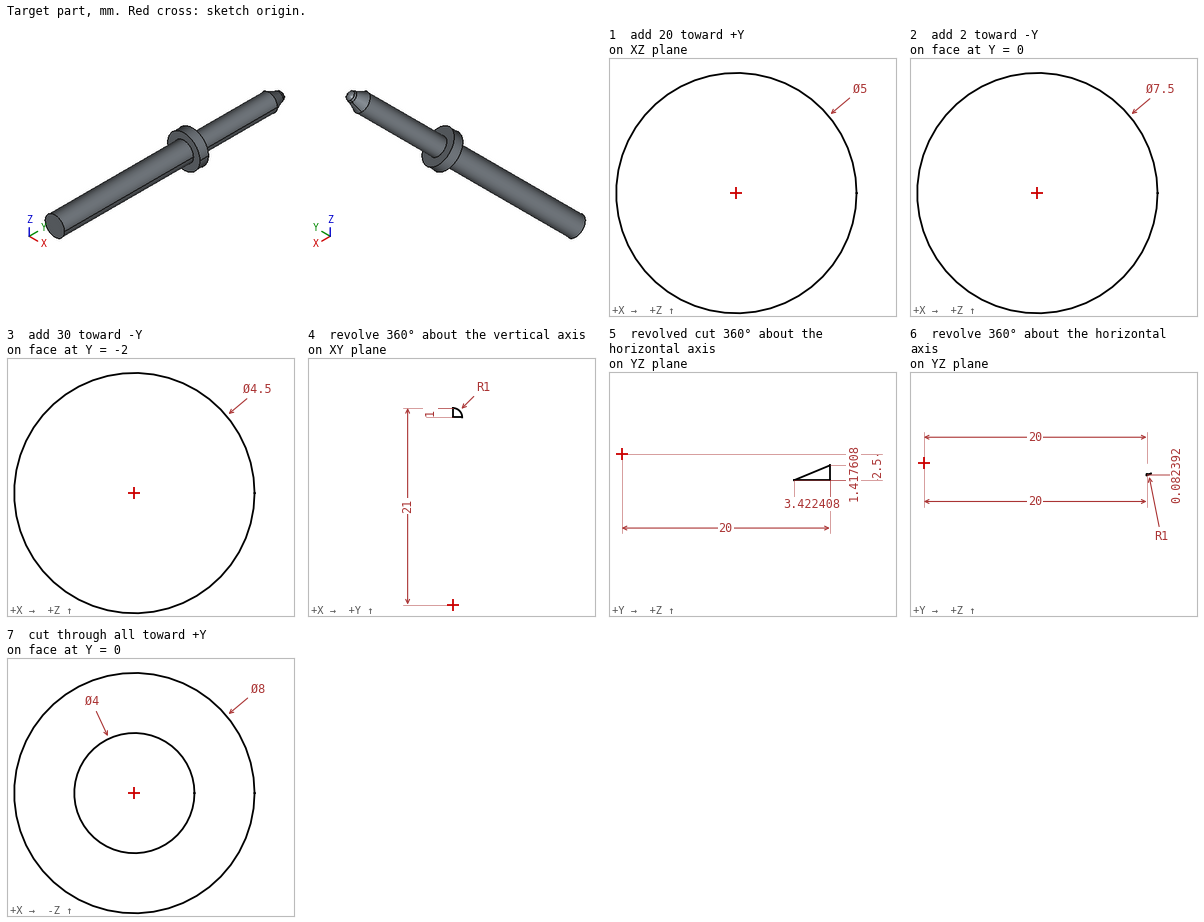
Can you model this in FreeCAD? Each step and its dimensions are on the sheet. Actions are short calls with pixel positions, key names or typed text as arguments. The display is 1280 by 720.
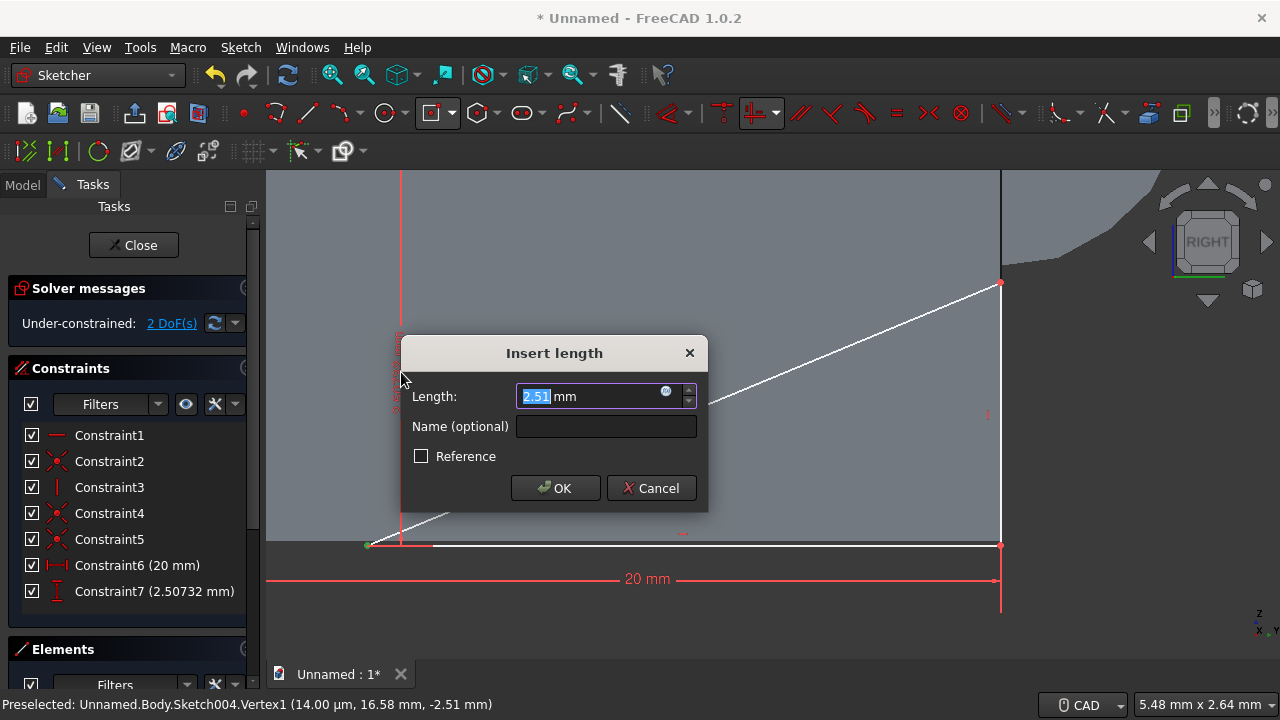
text(2.5)
key(Return)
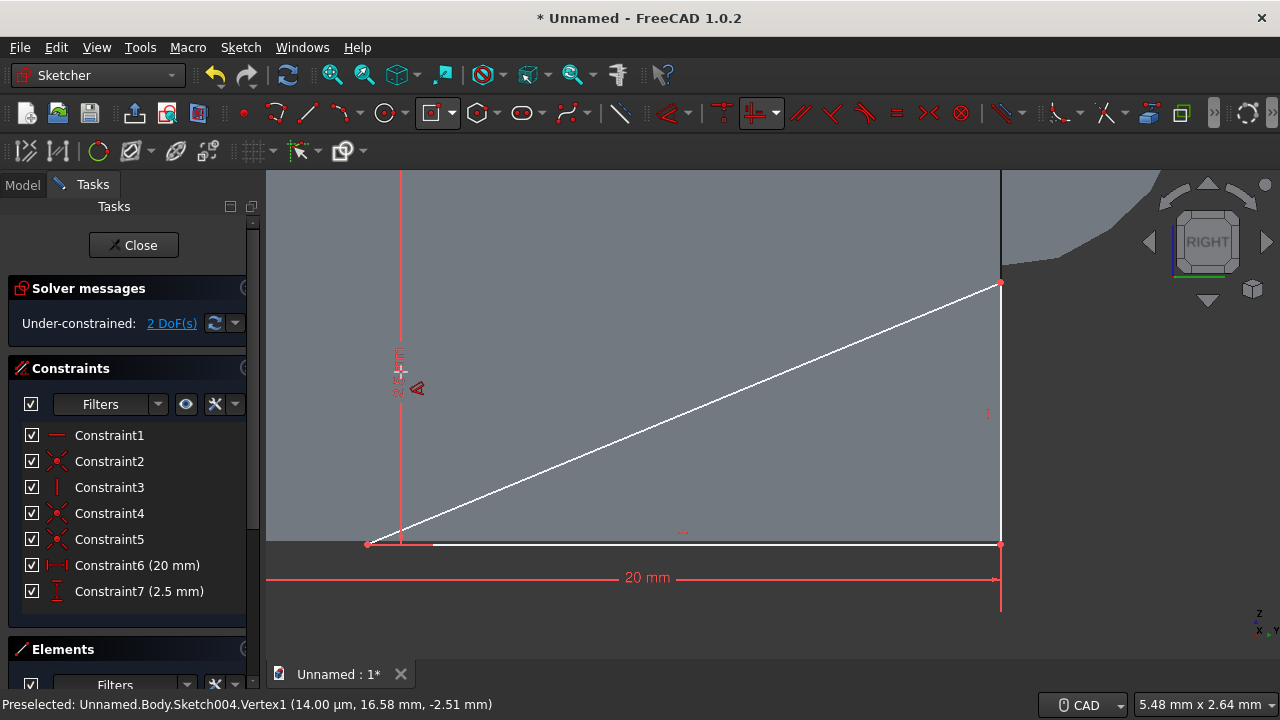
click(557, 545)
click(538, 579)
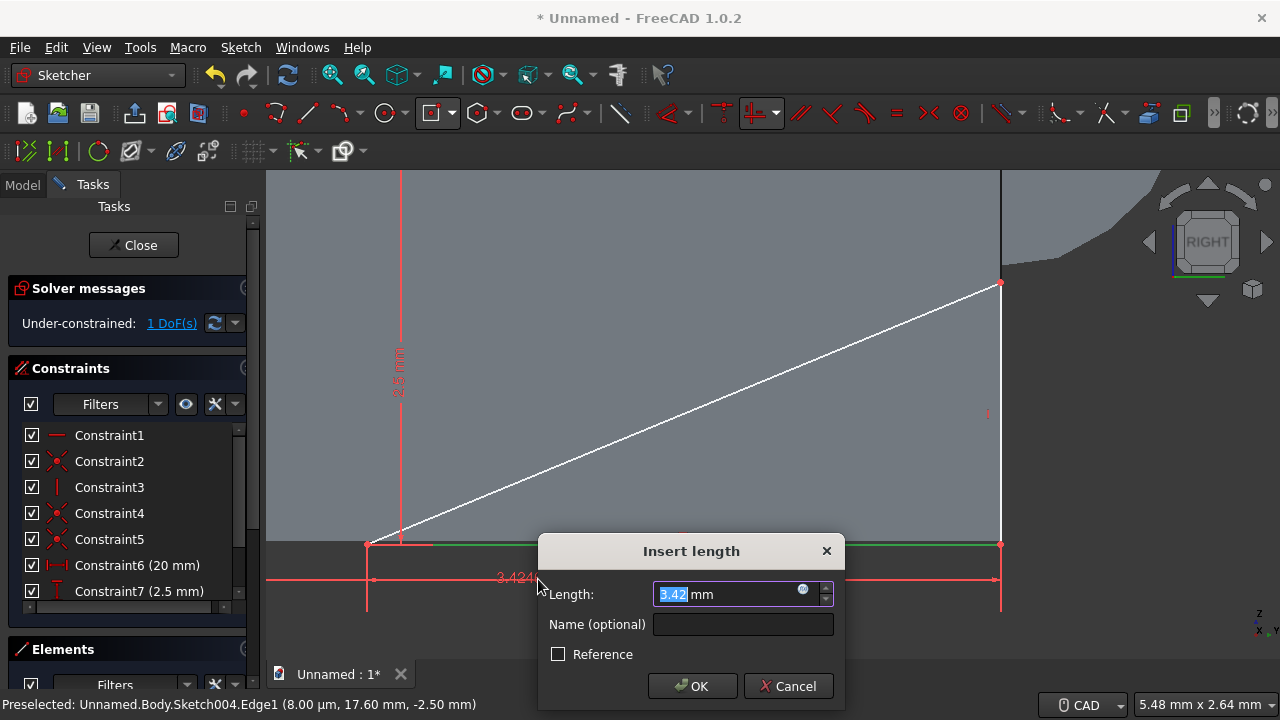
text(3.422408)
key(Return)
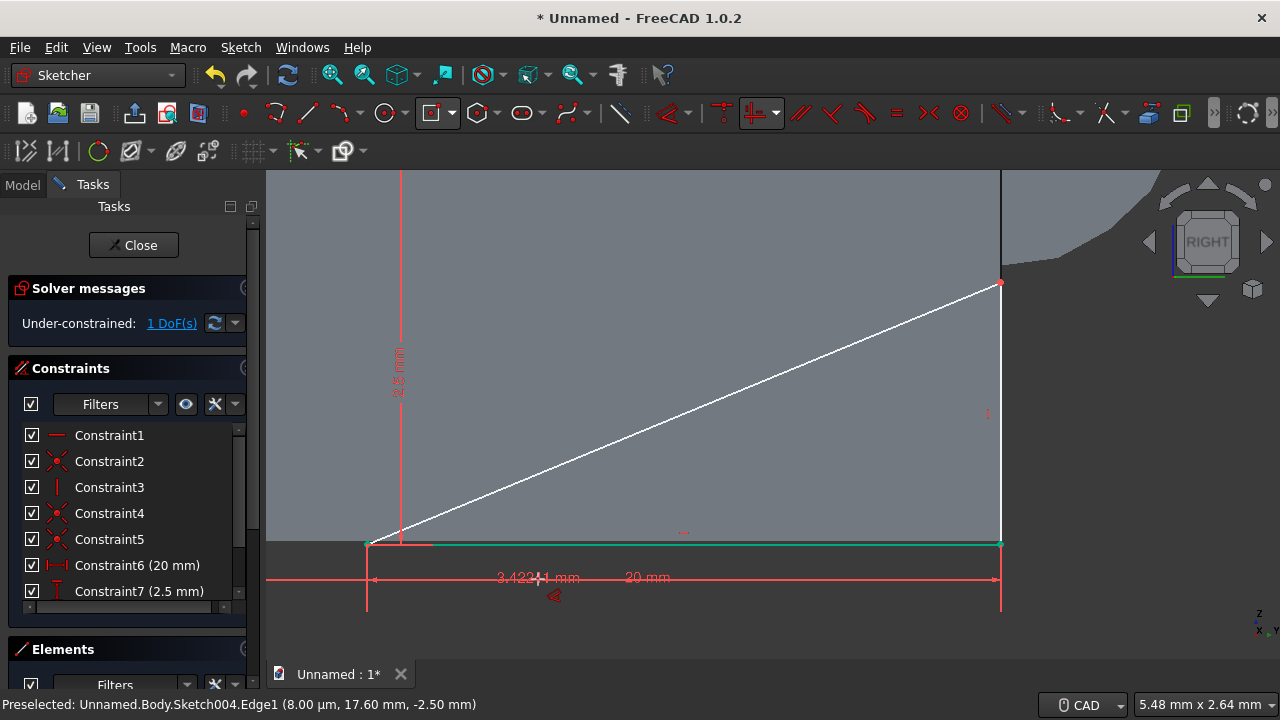
click(1001, 466)
click(1035, 414)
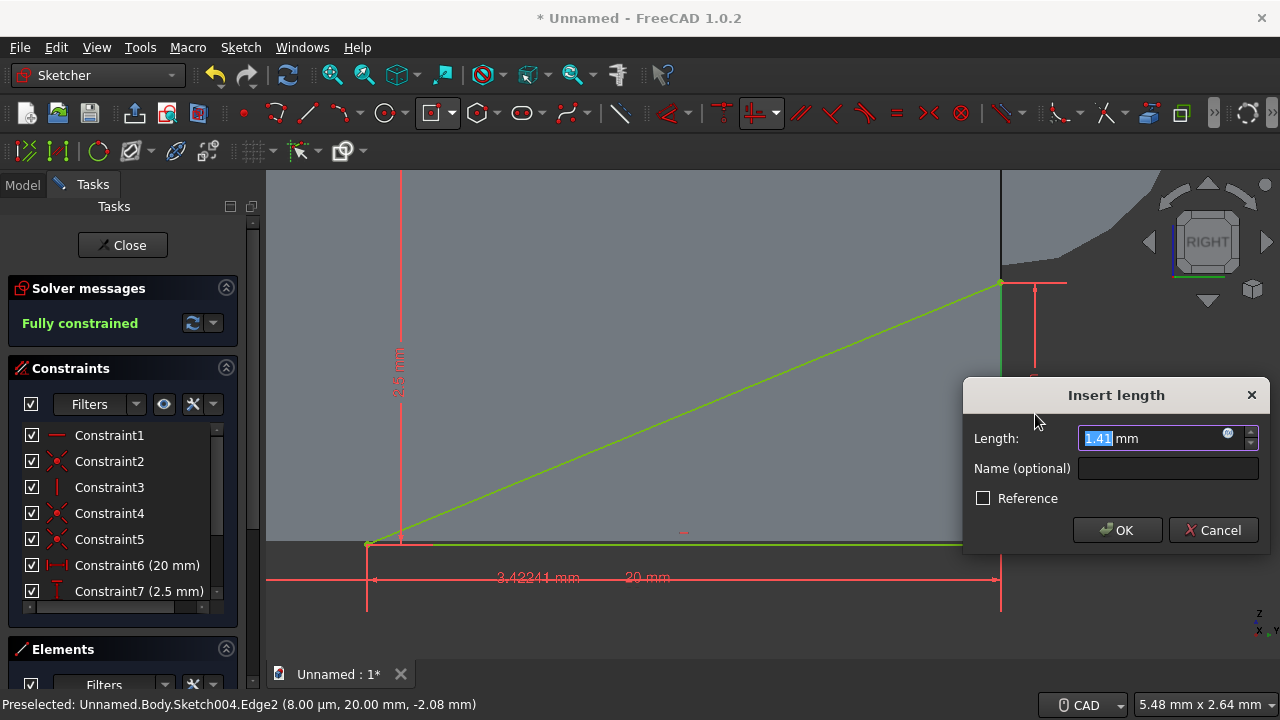
text(1.417608)
key(Return)
key(Escape)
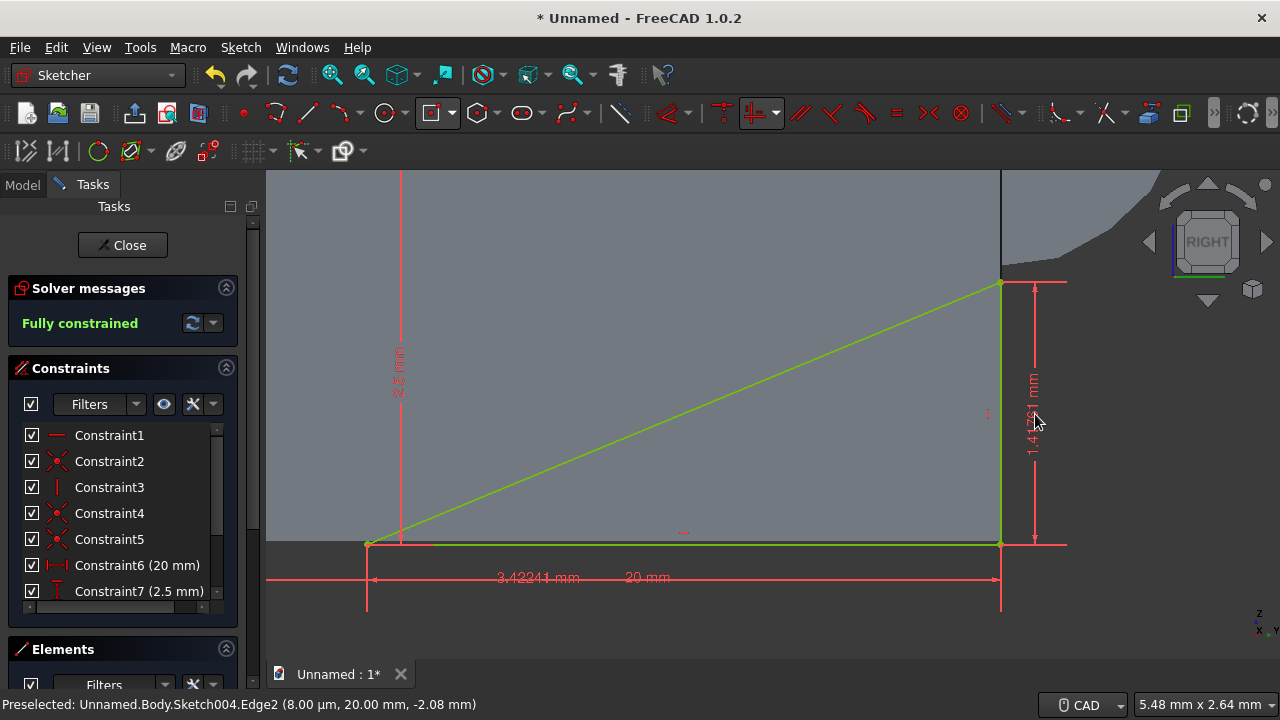
click(123, 245)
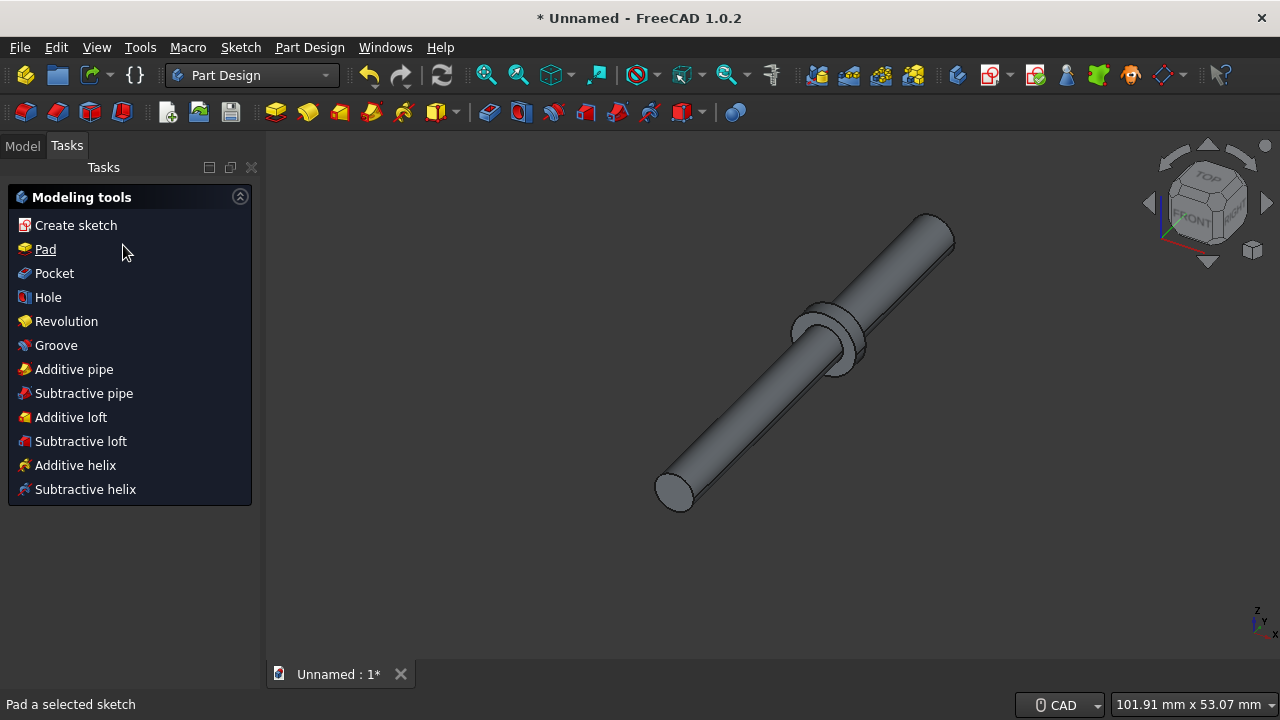
click(554, 112)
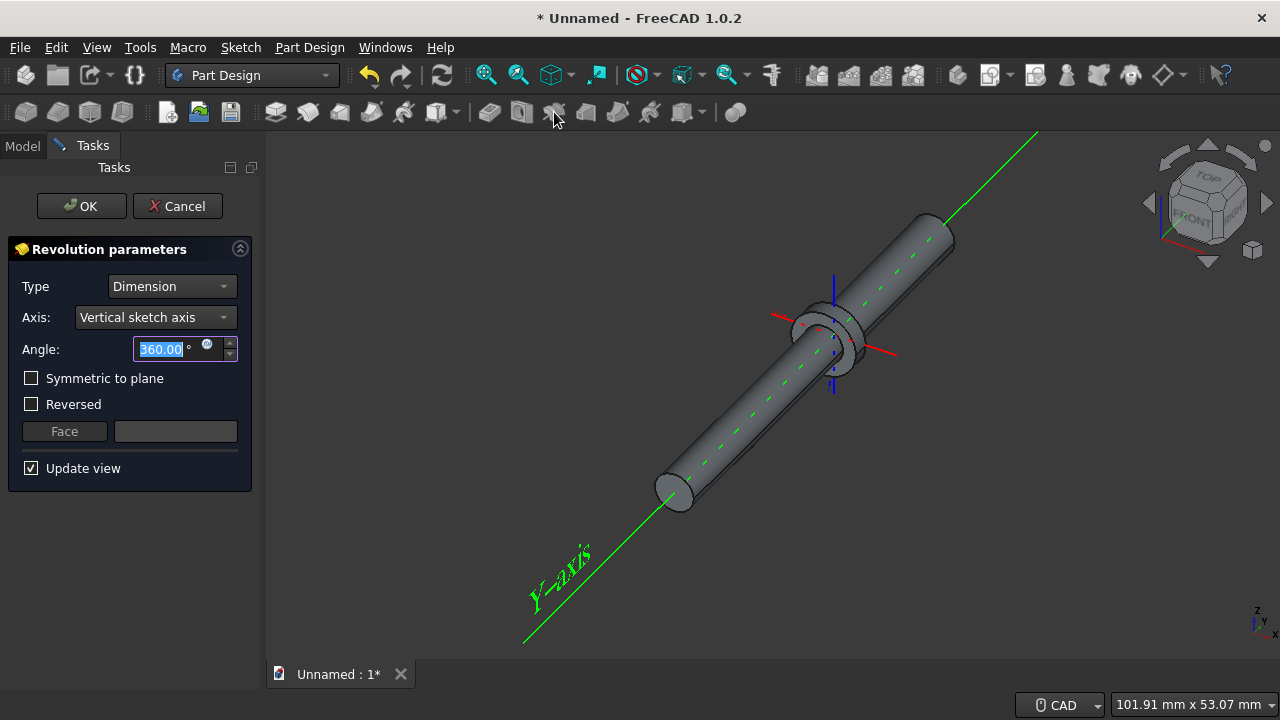
click(156, 318)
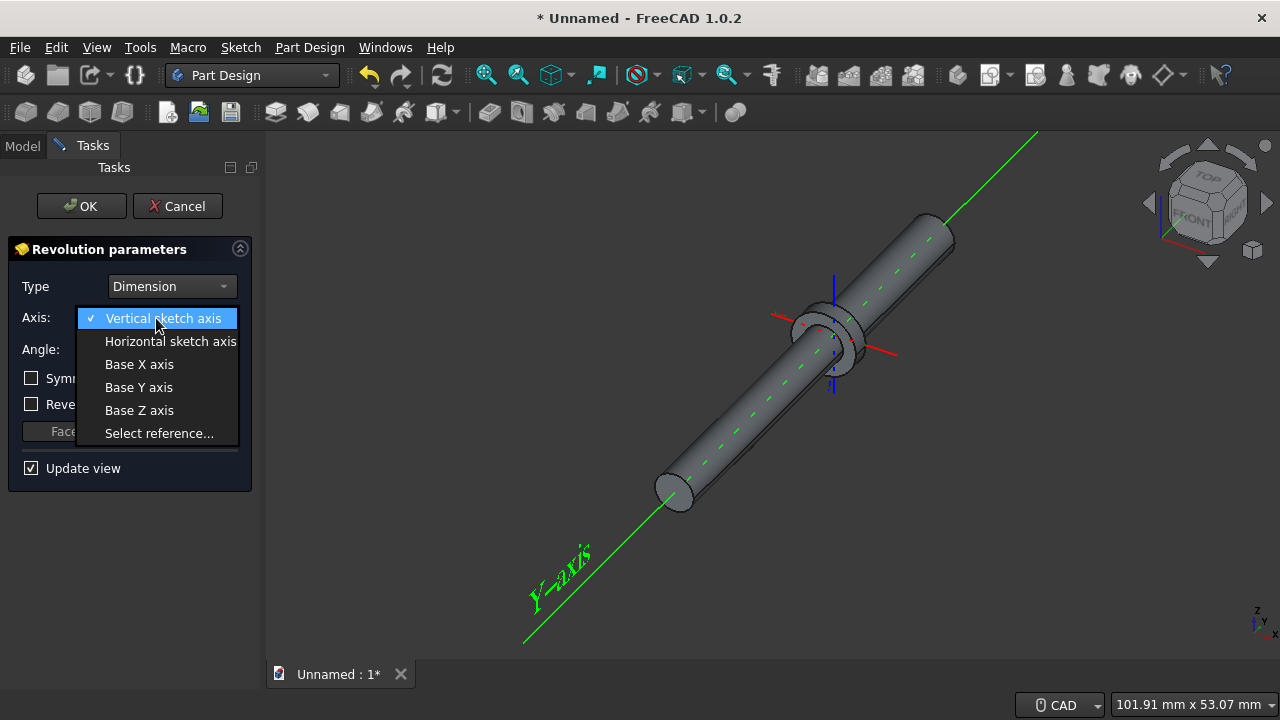
click(156, 342)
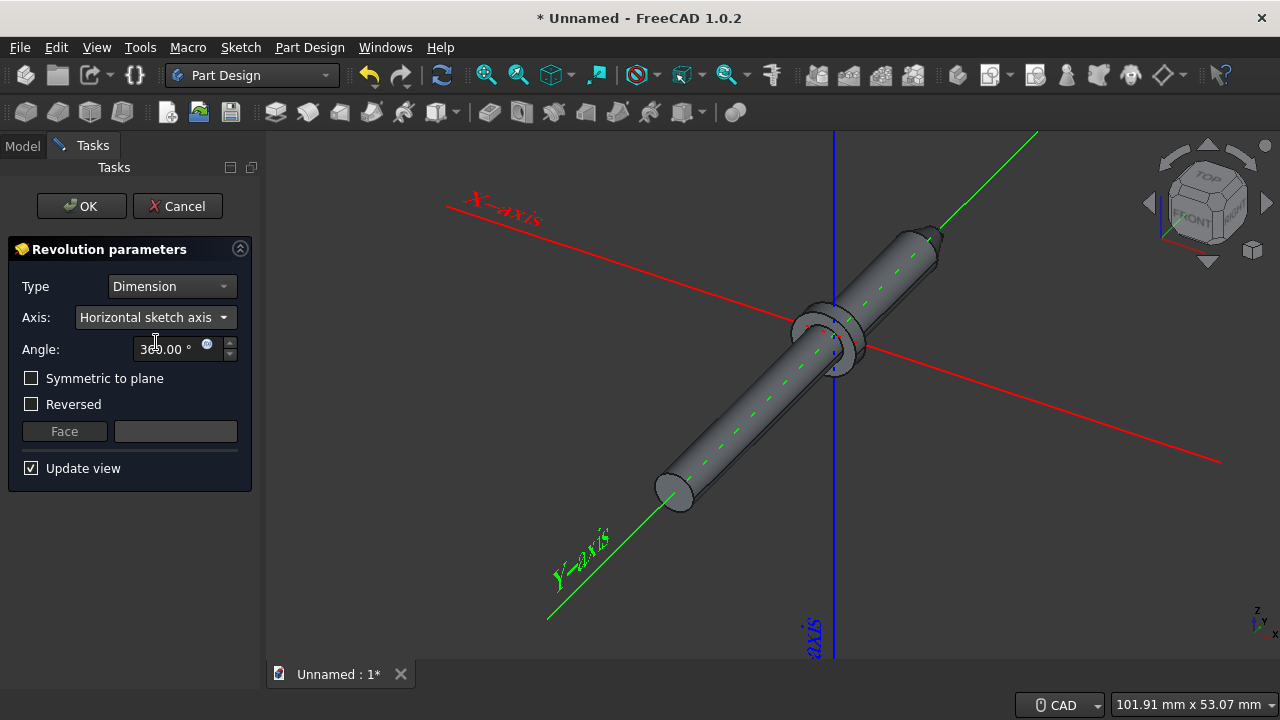
click(82, 206)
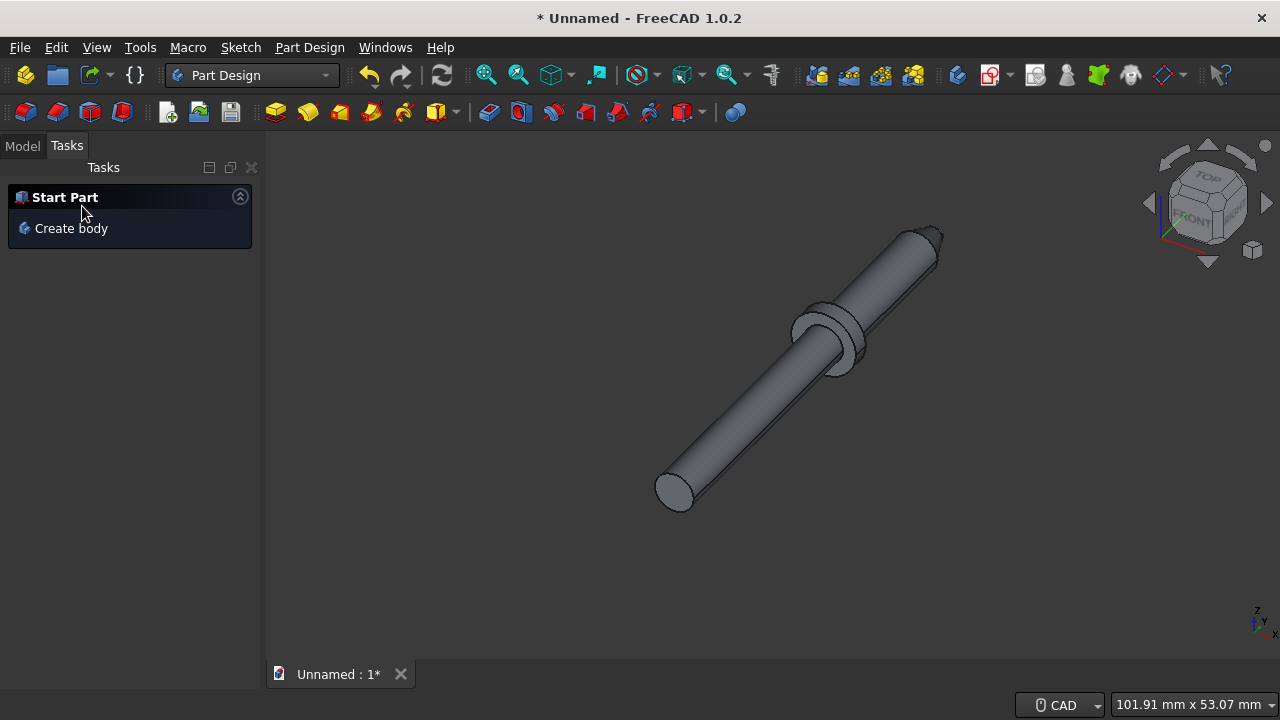
click(990, 76)